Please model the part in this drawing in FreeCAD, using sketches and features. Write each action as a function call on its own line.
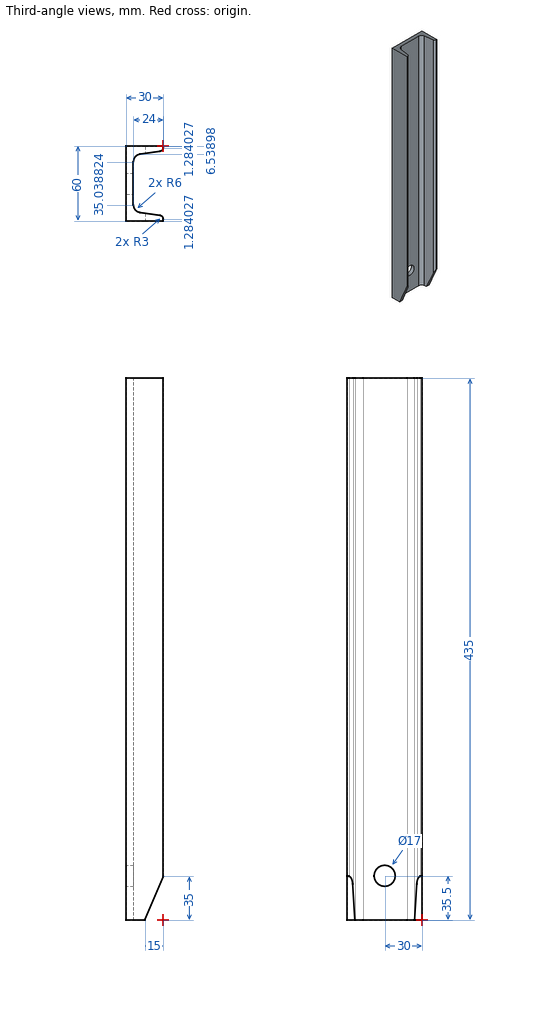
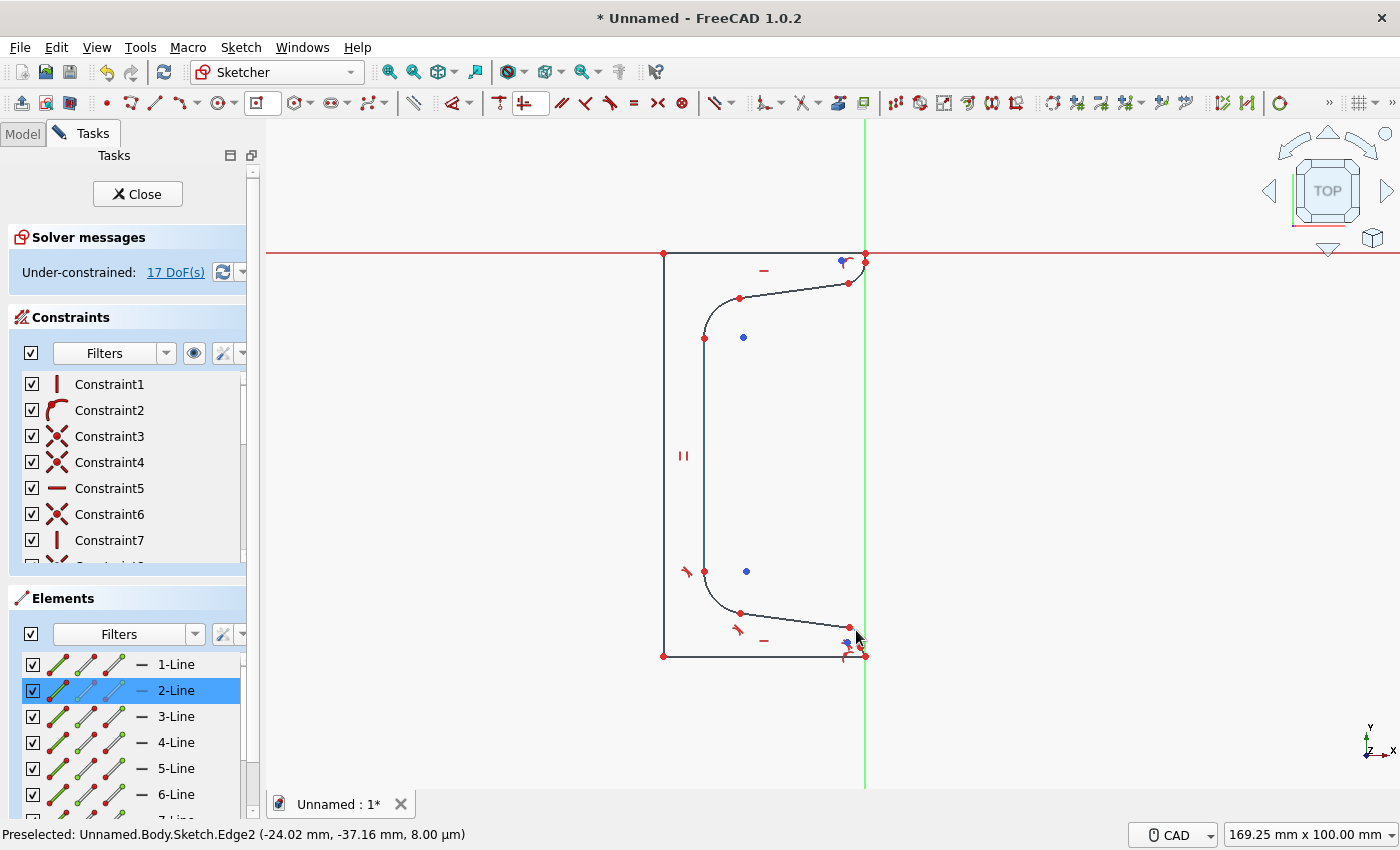
click(723, 304)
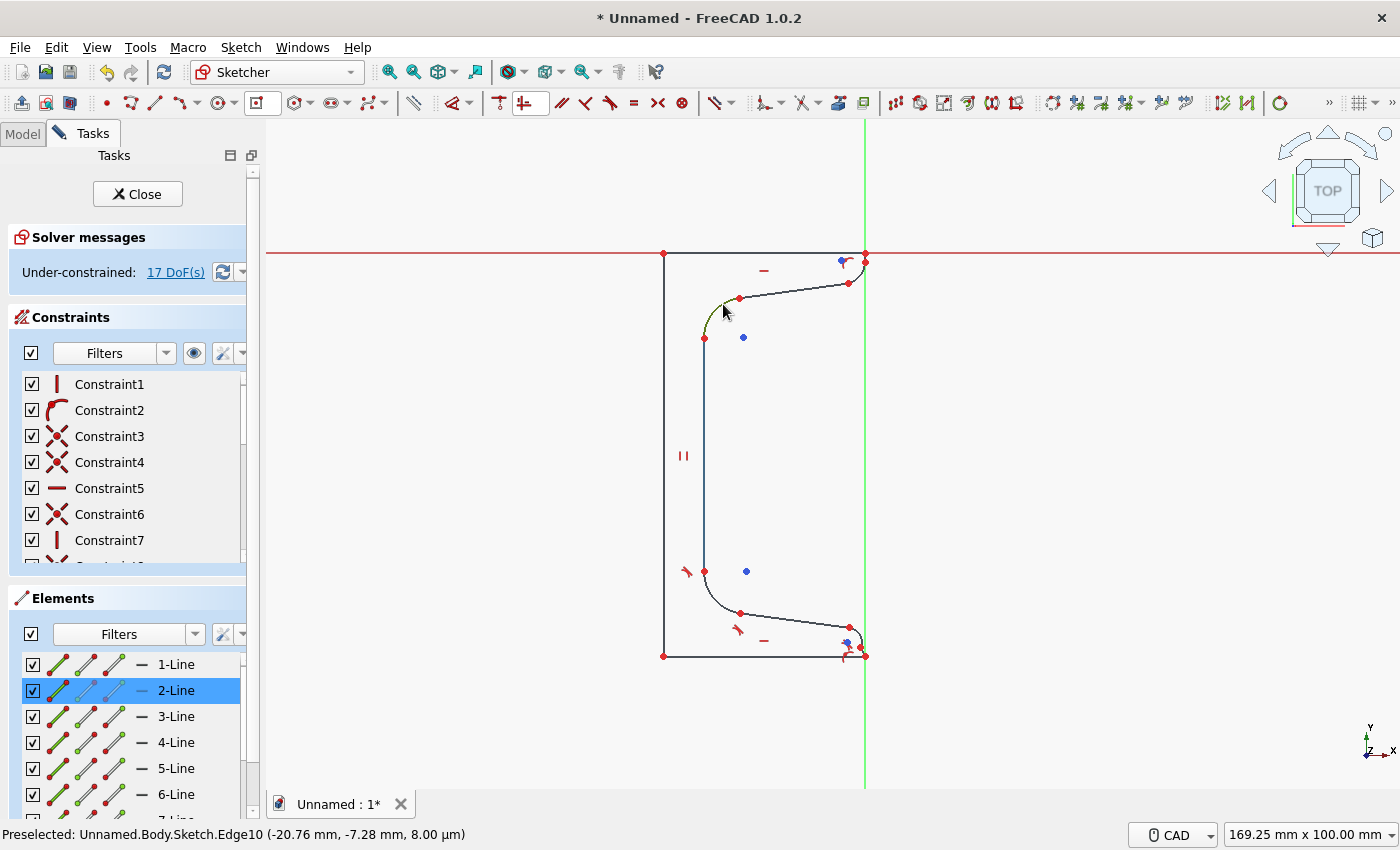
click(610, 104)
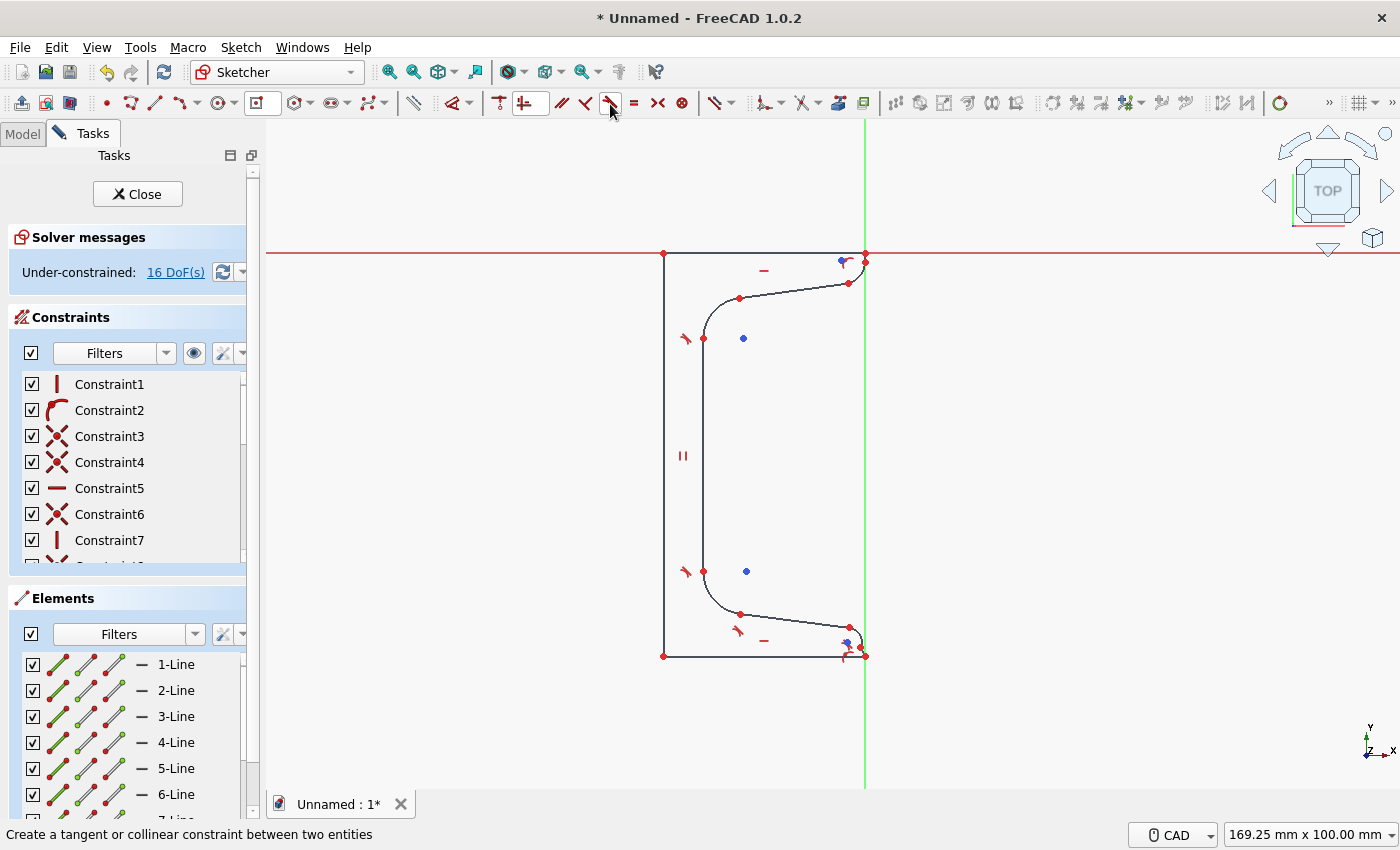
click(772, 294)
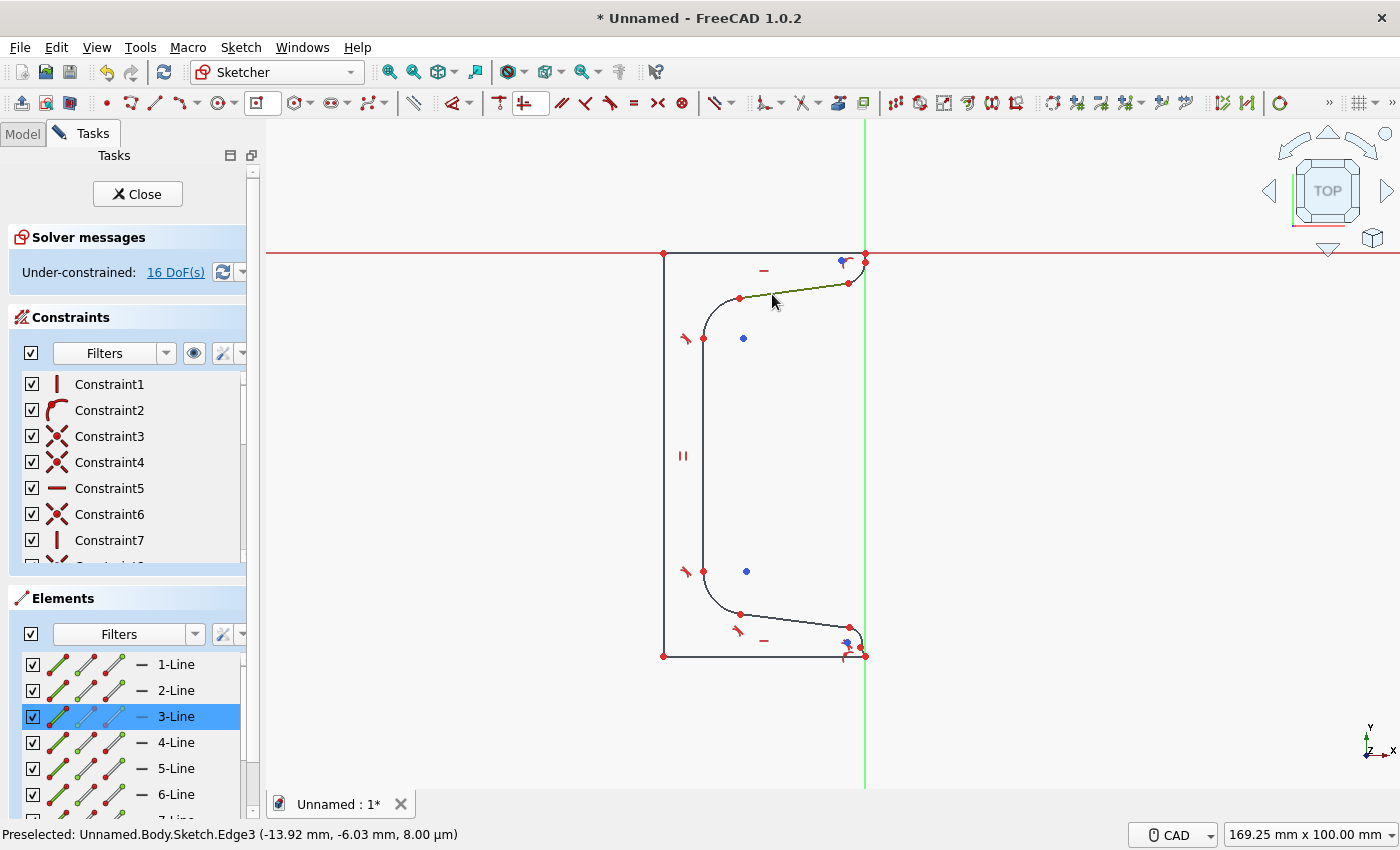
click(723, 304)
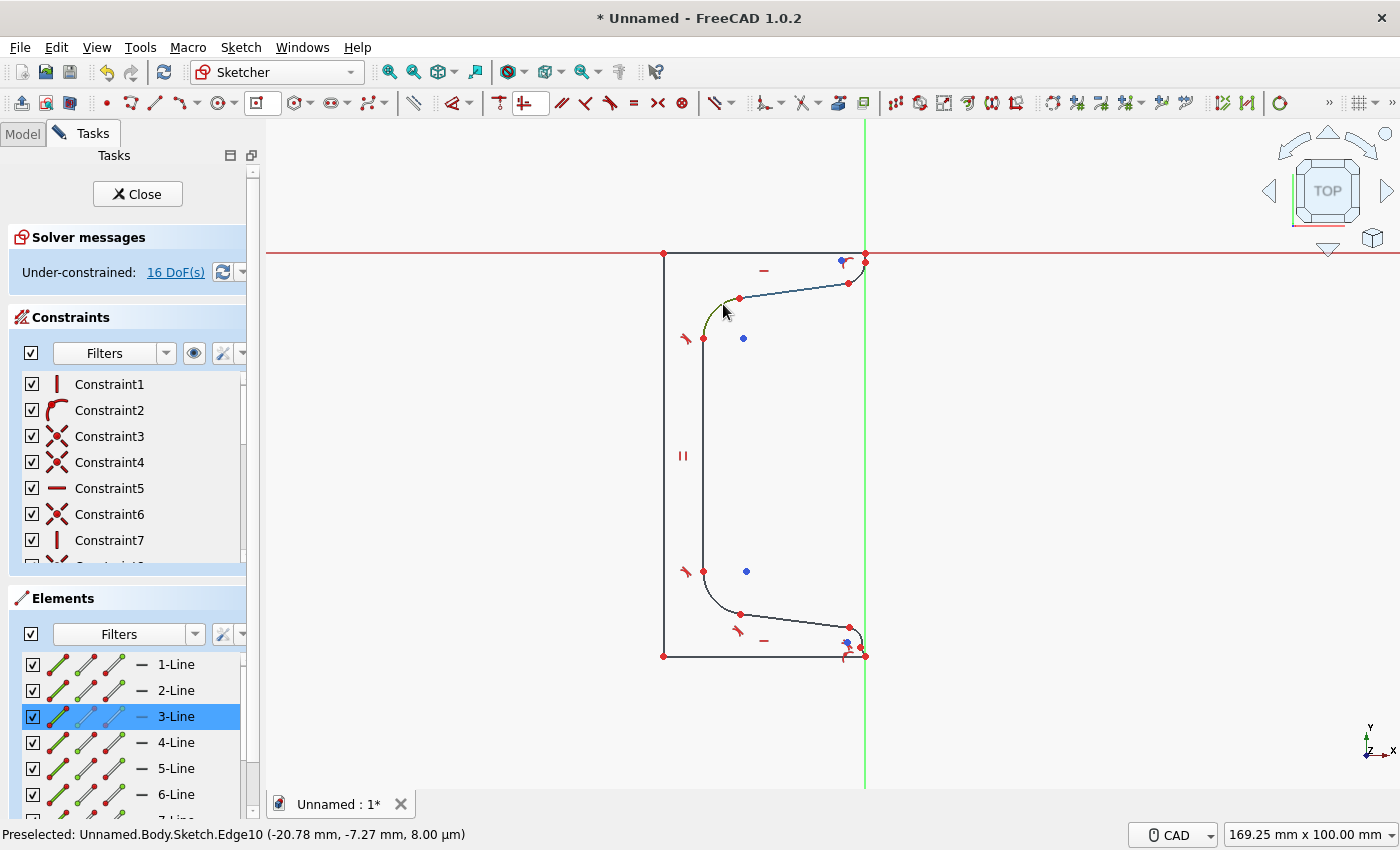
click(610, 104)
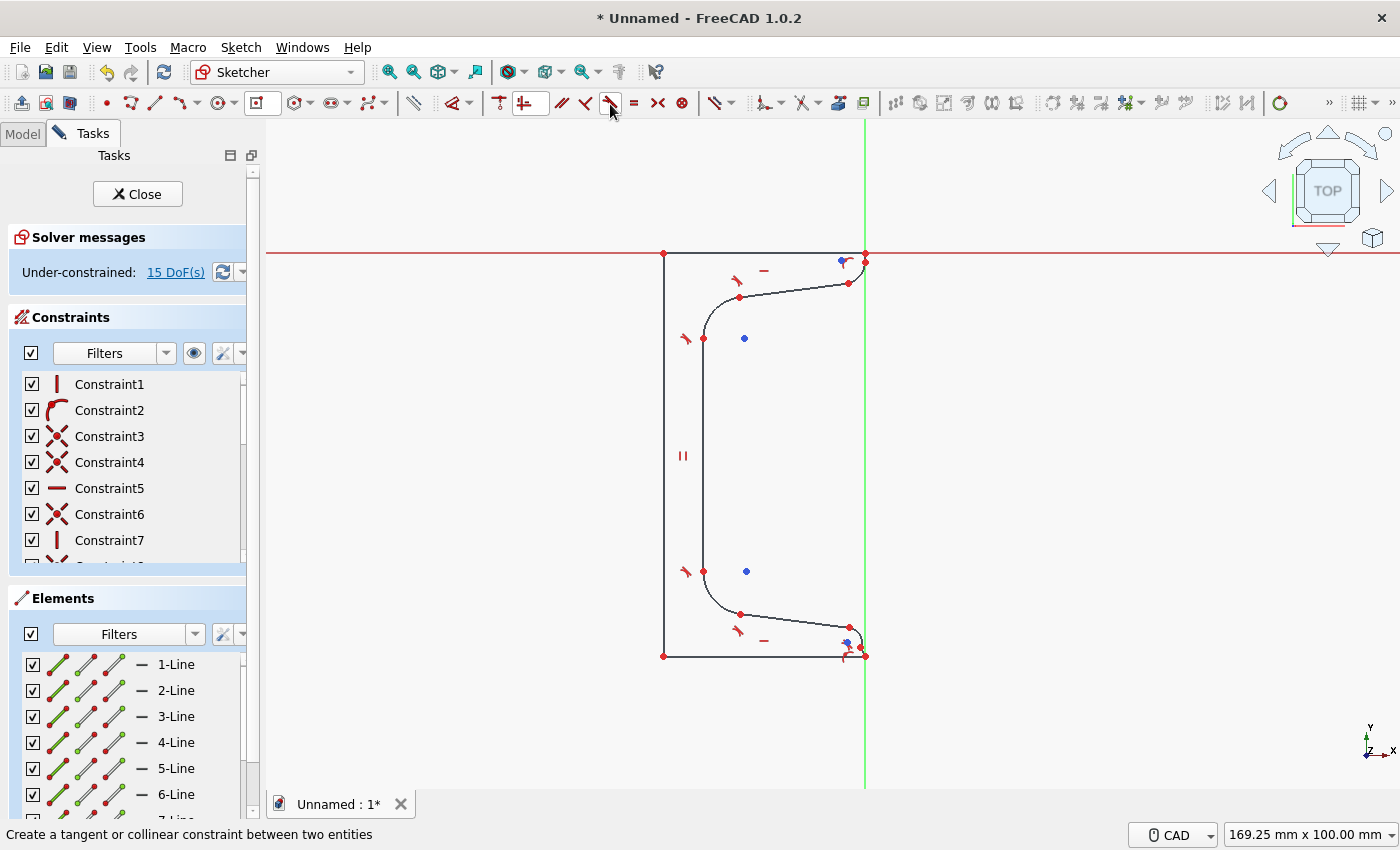
click(772, 293)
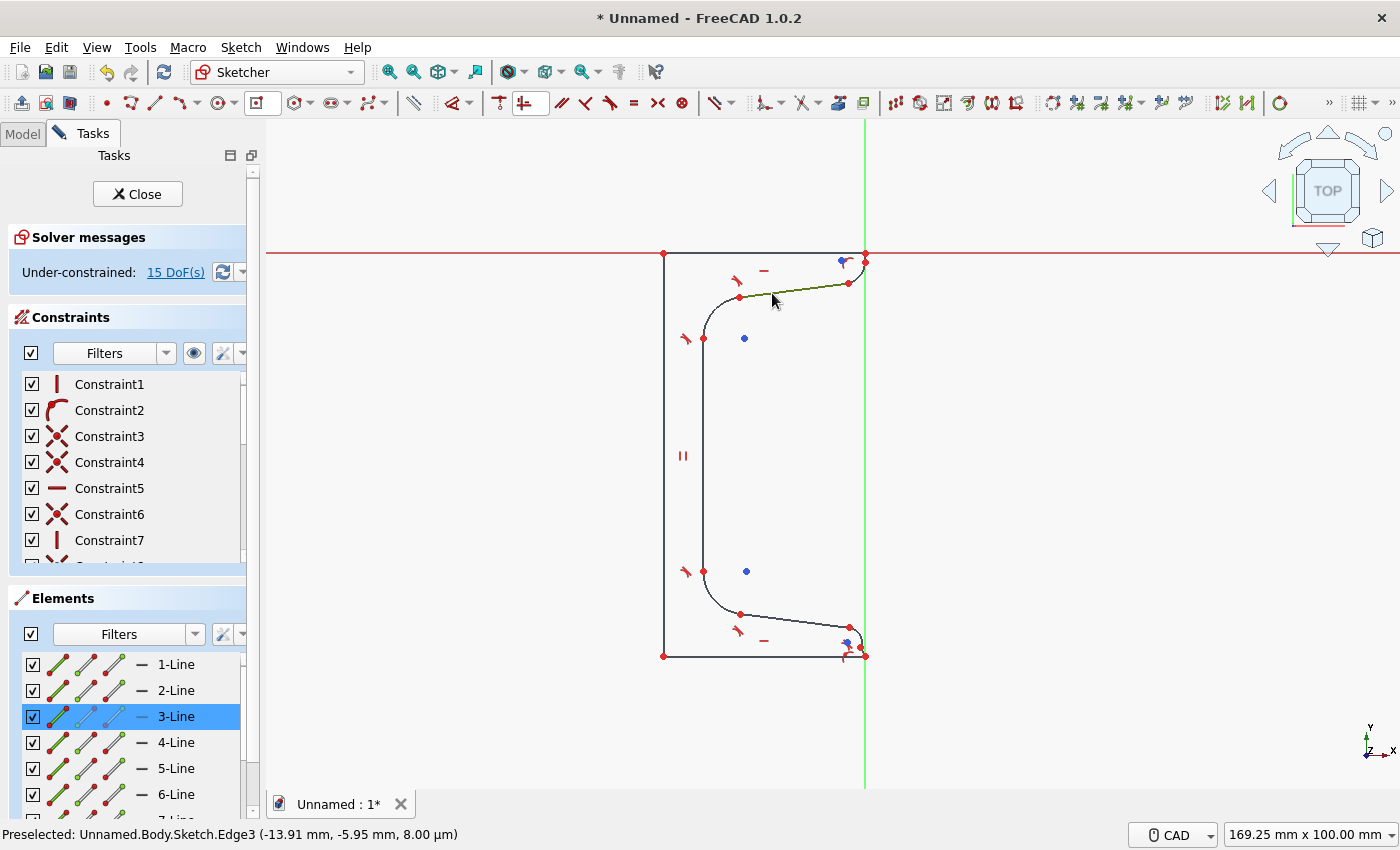
scroll(863, 271, up, 3)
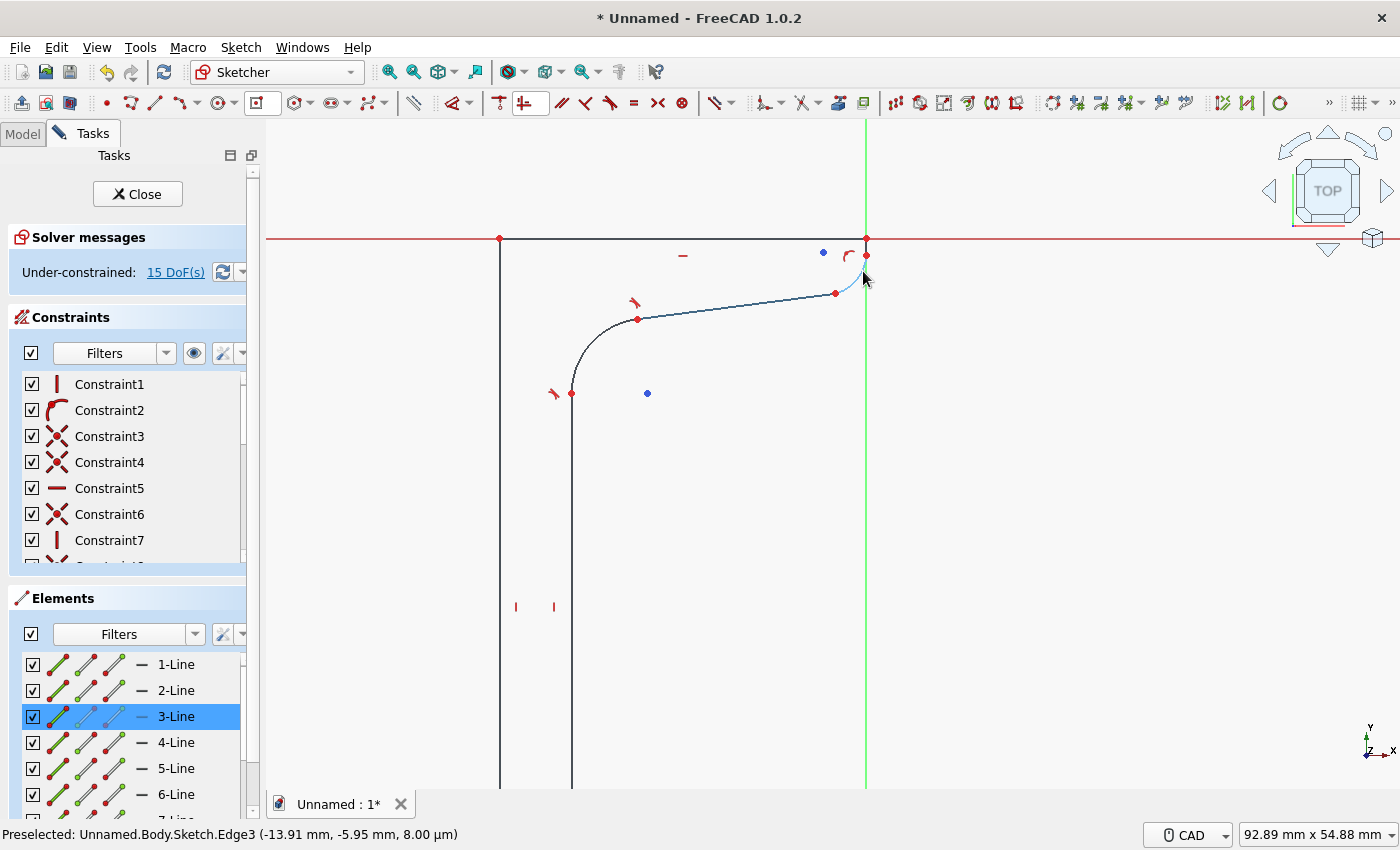
click(863, 270)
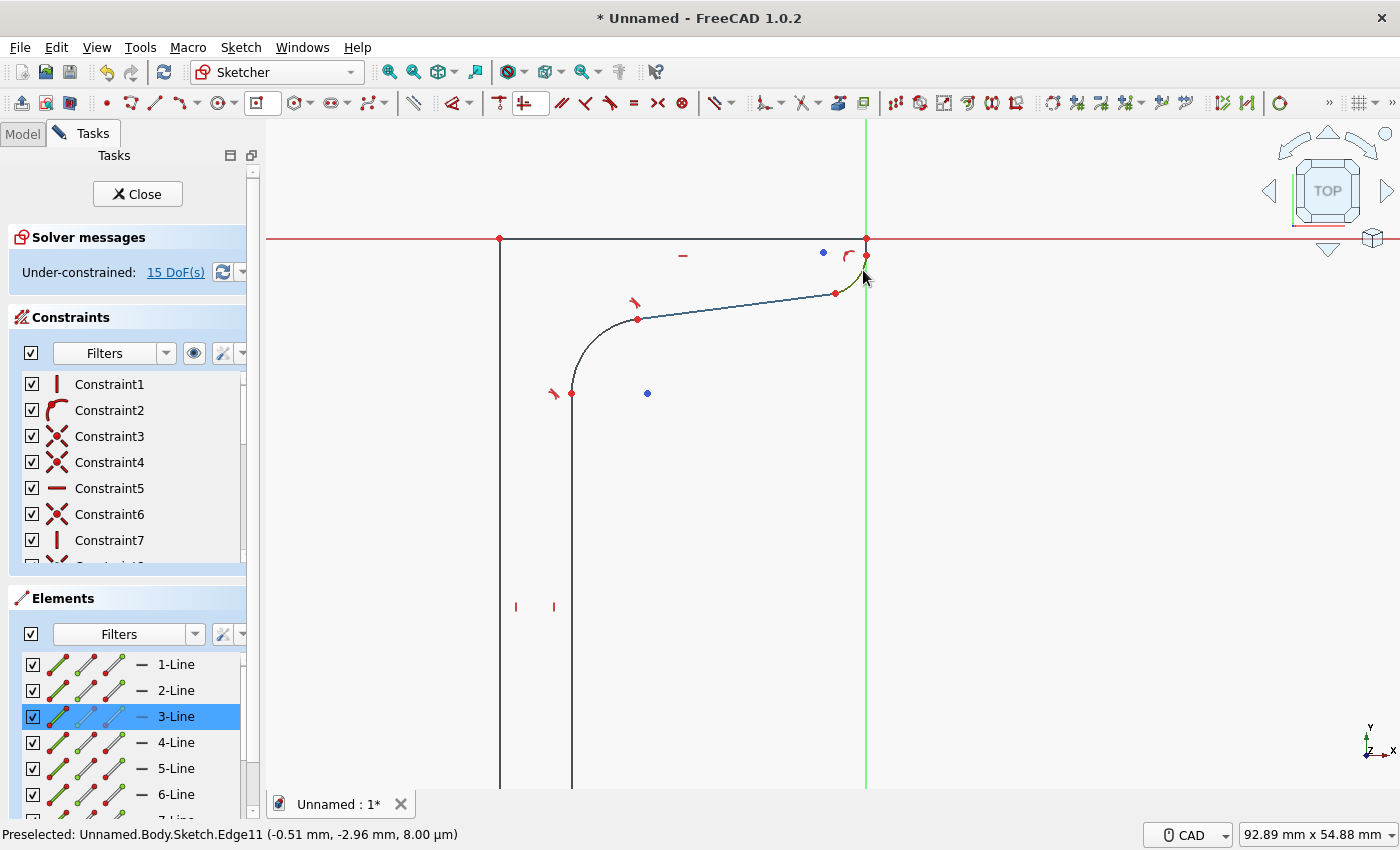
click(610, 104)